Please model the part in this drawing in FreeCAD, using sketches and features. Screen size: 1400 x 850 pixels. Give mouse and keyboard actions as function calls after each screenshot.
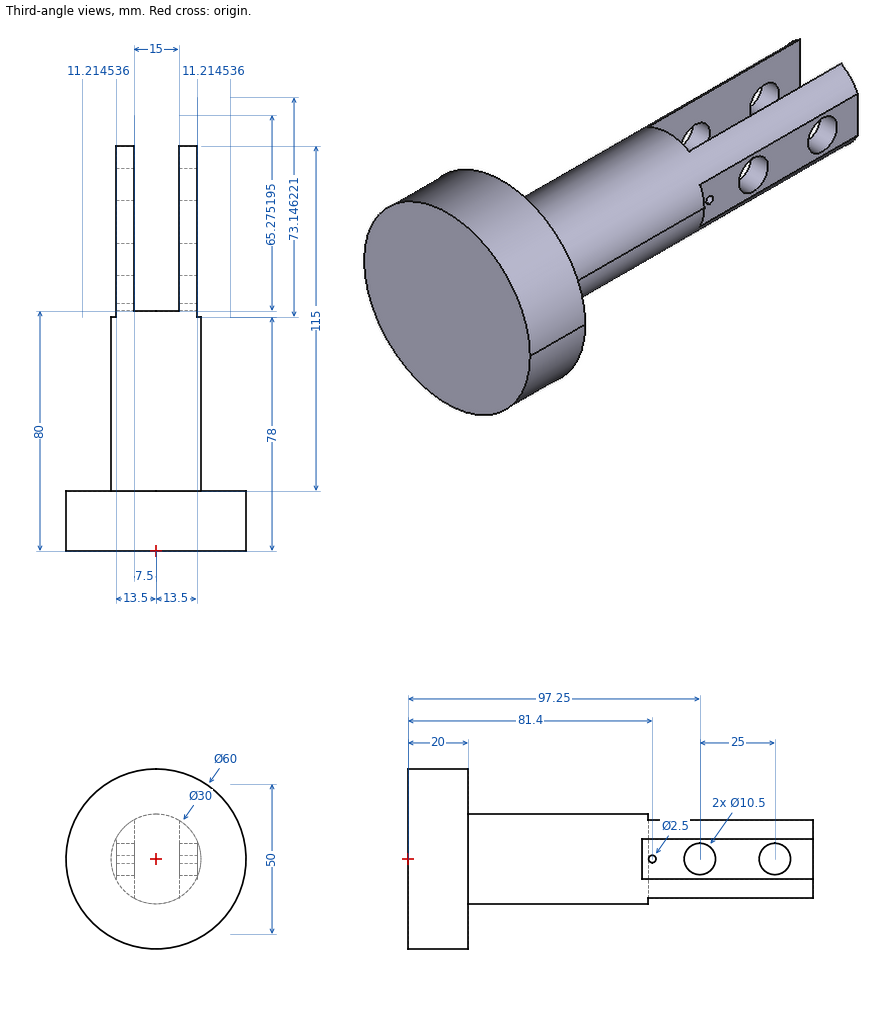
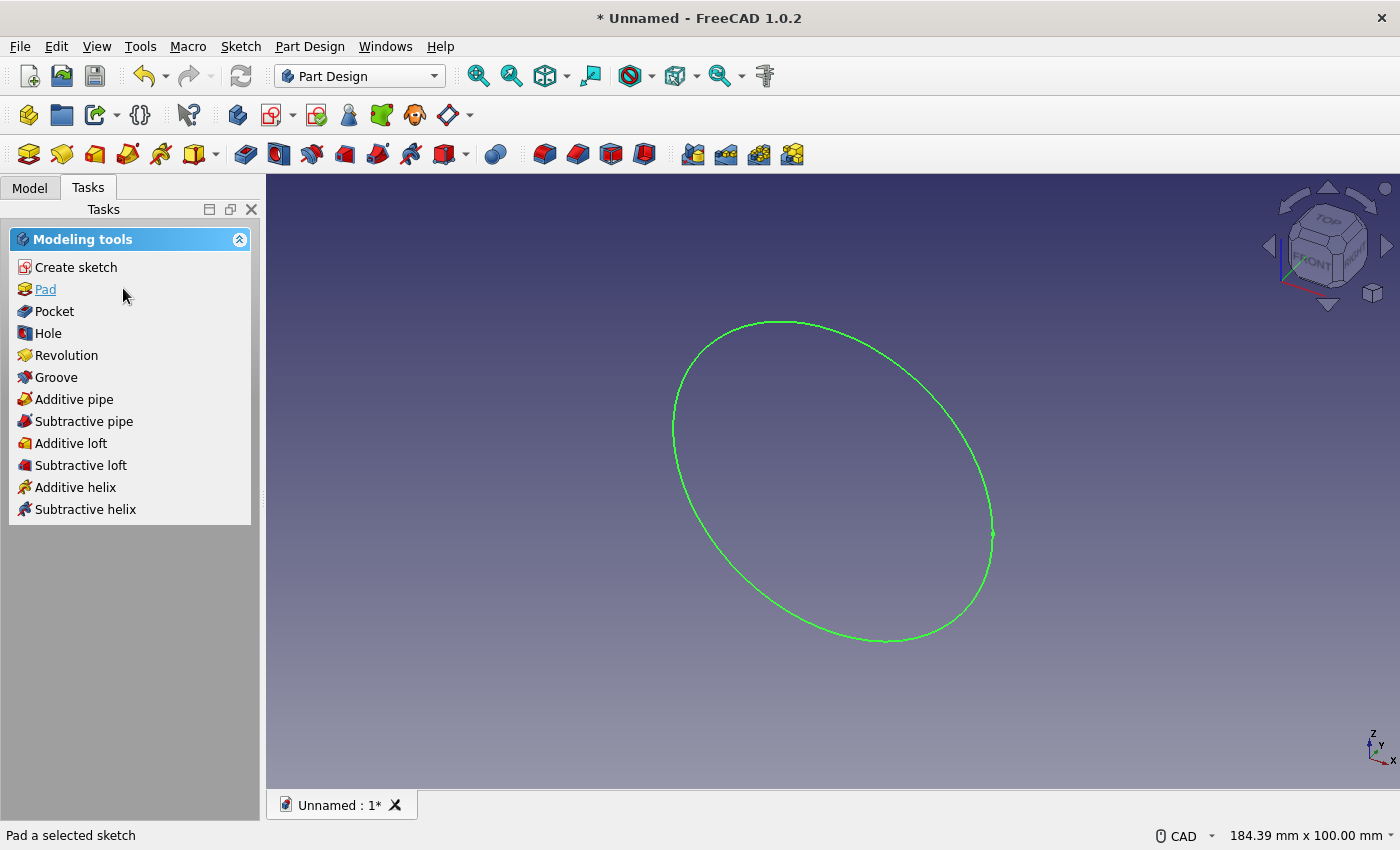
click(29, 154)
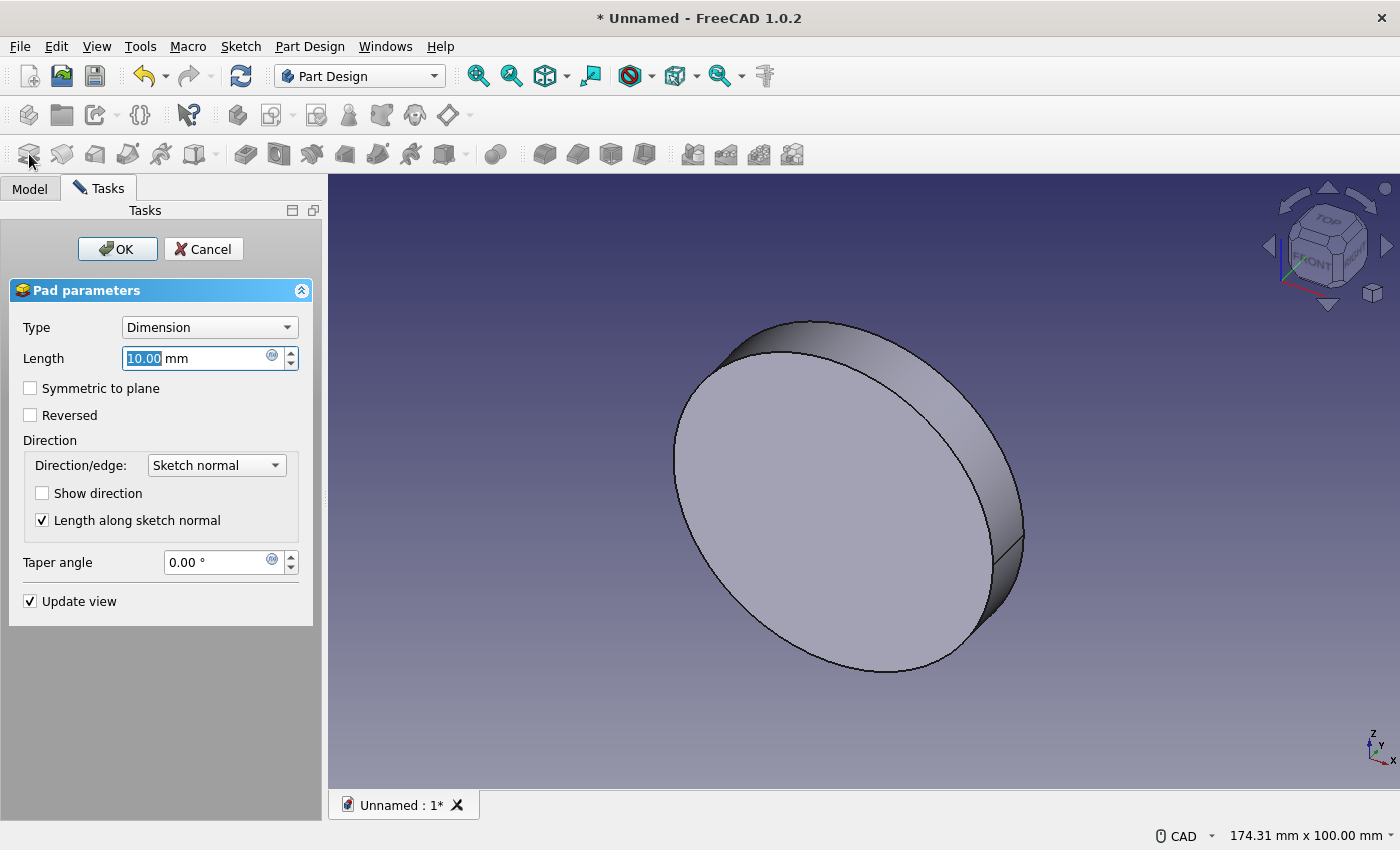
text(20)
key(Tab)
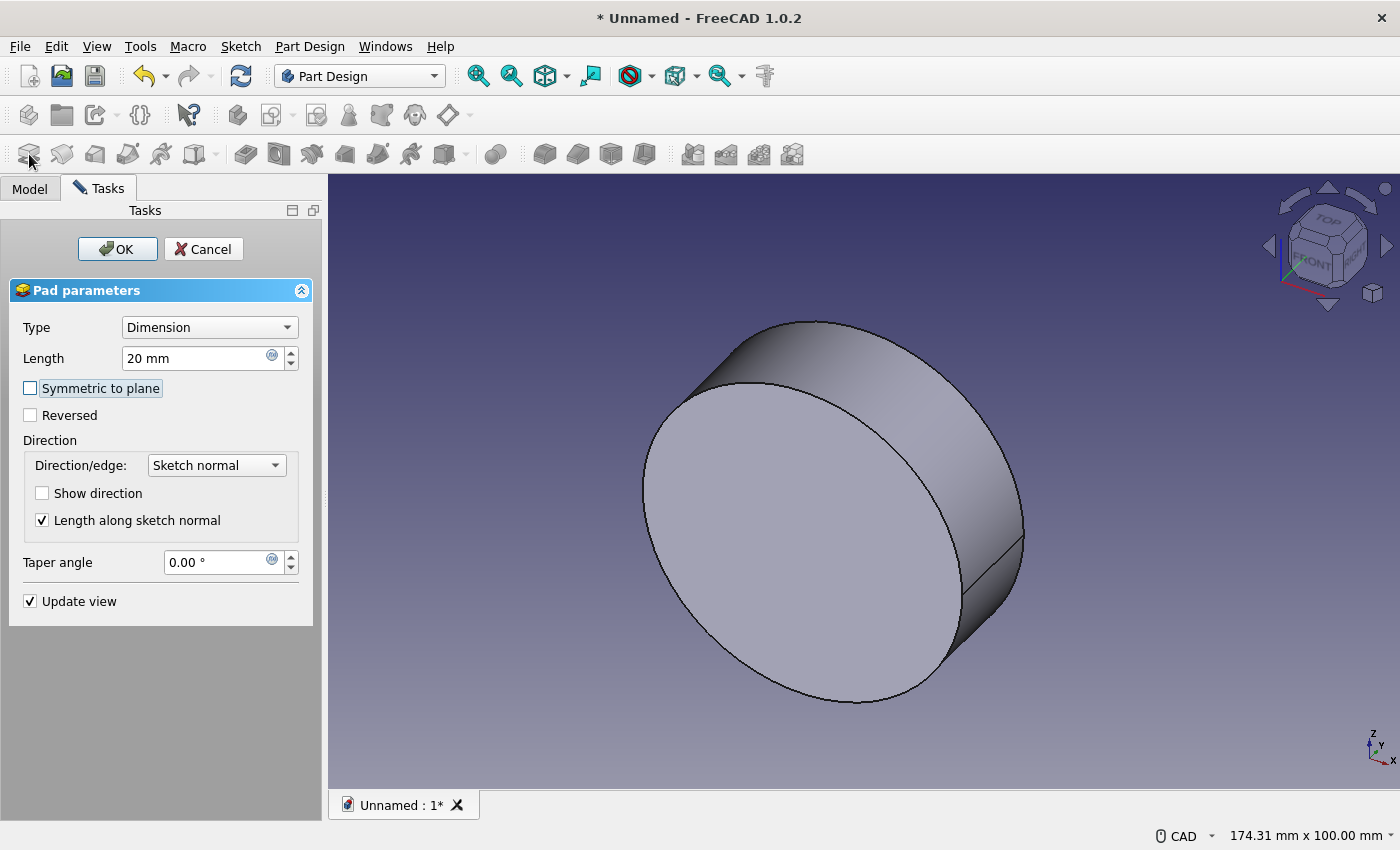
click(31, 415)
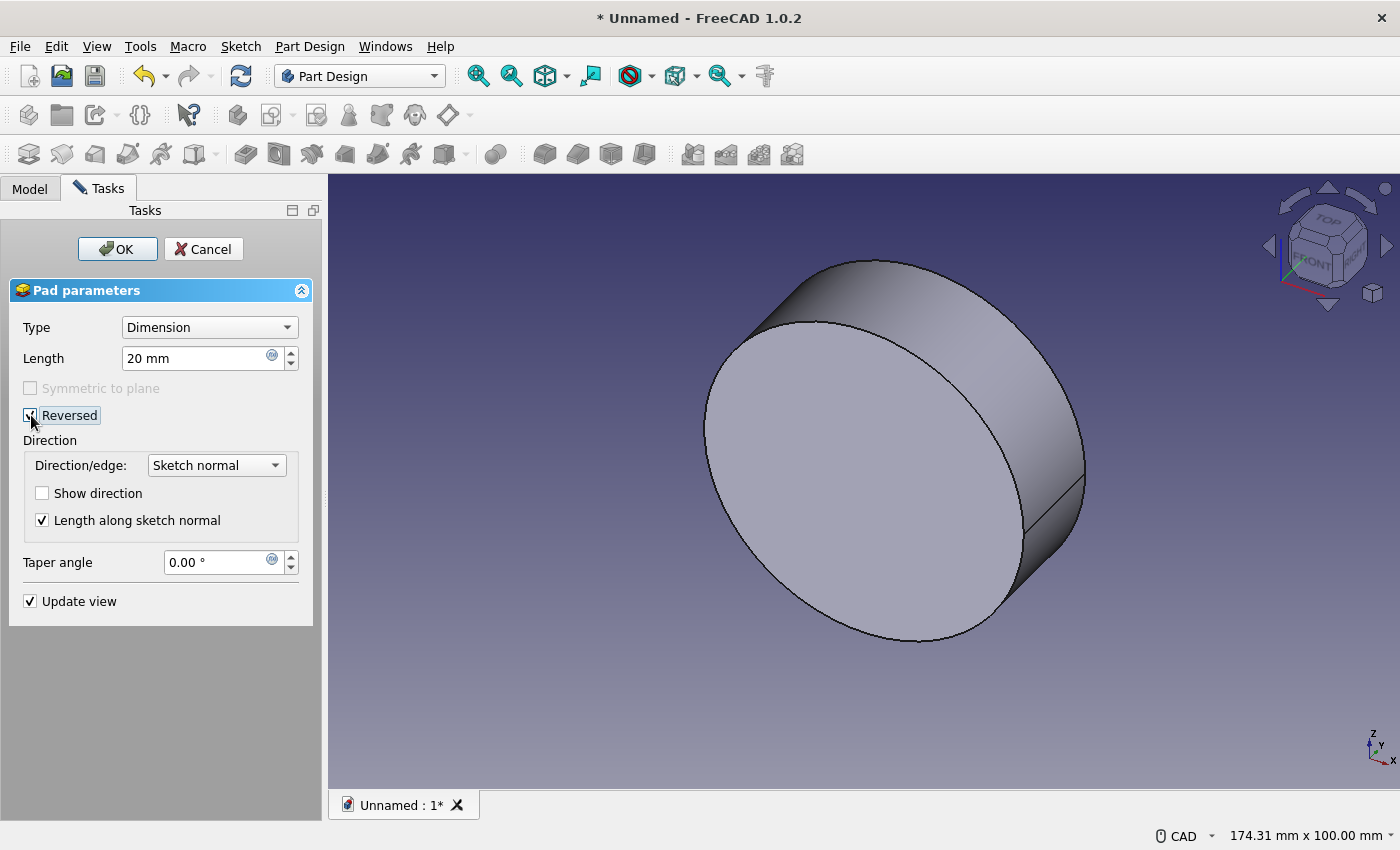
click(118, 249)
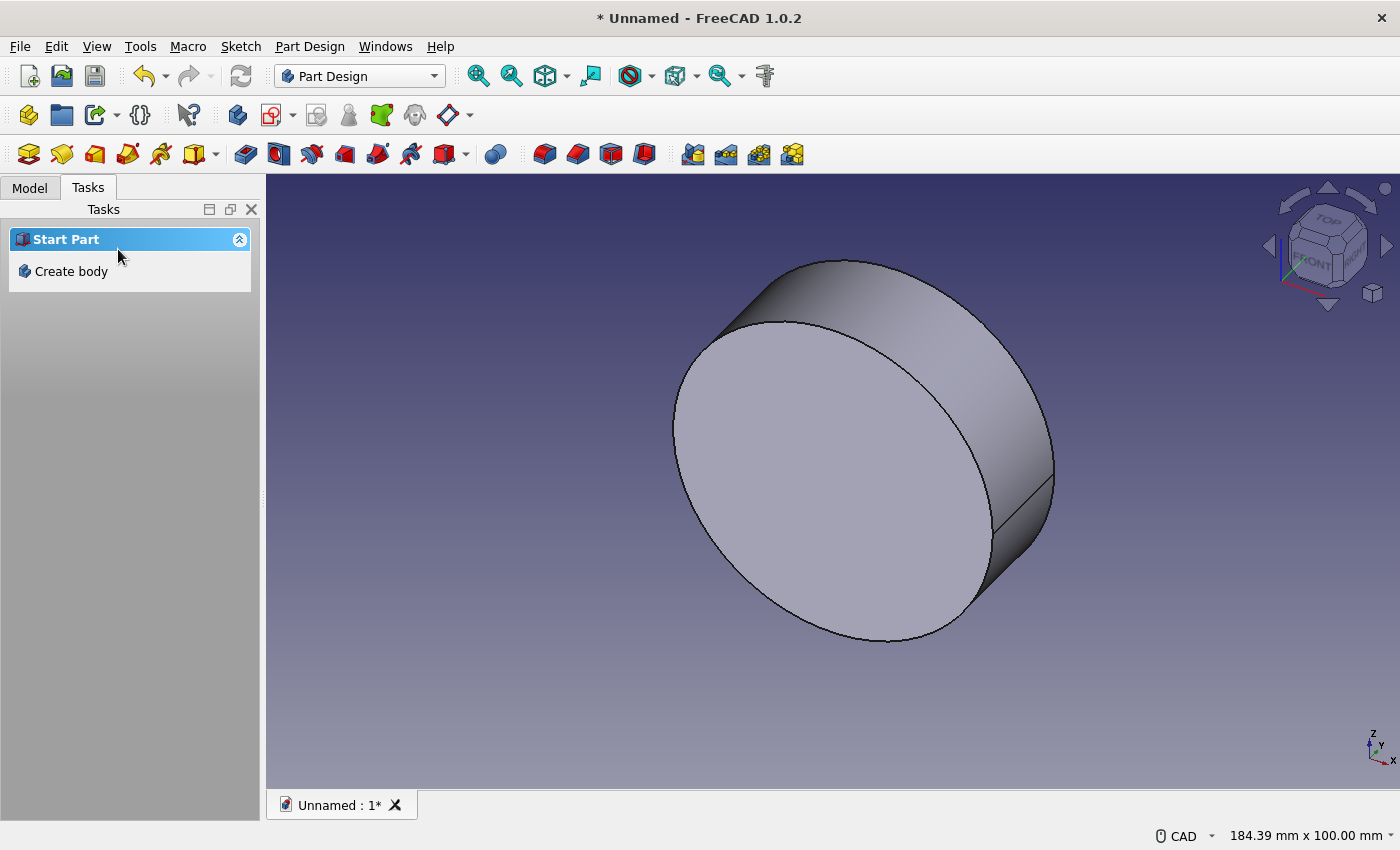
key(4)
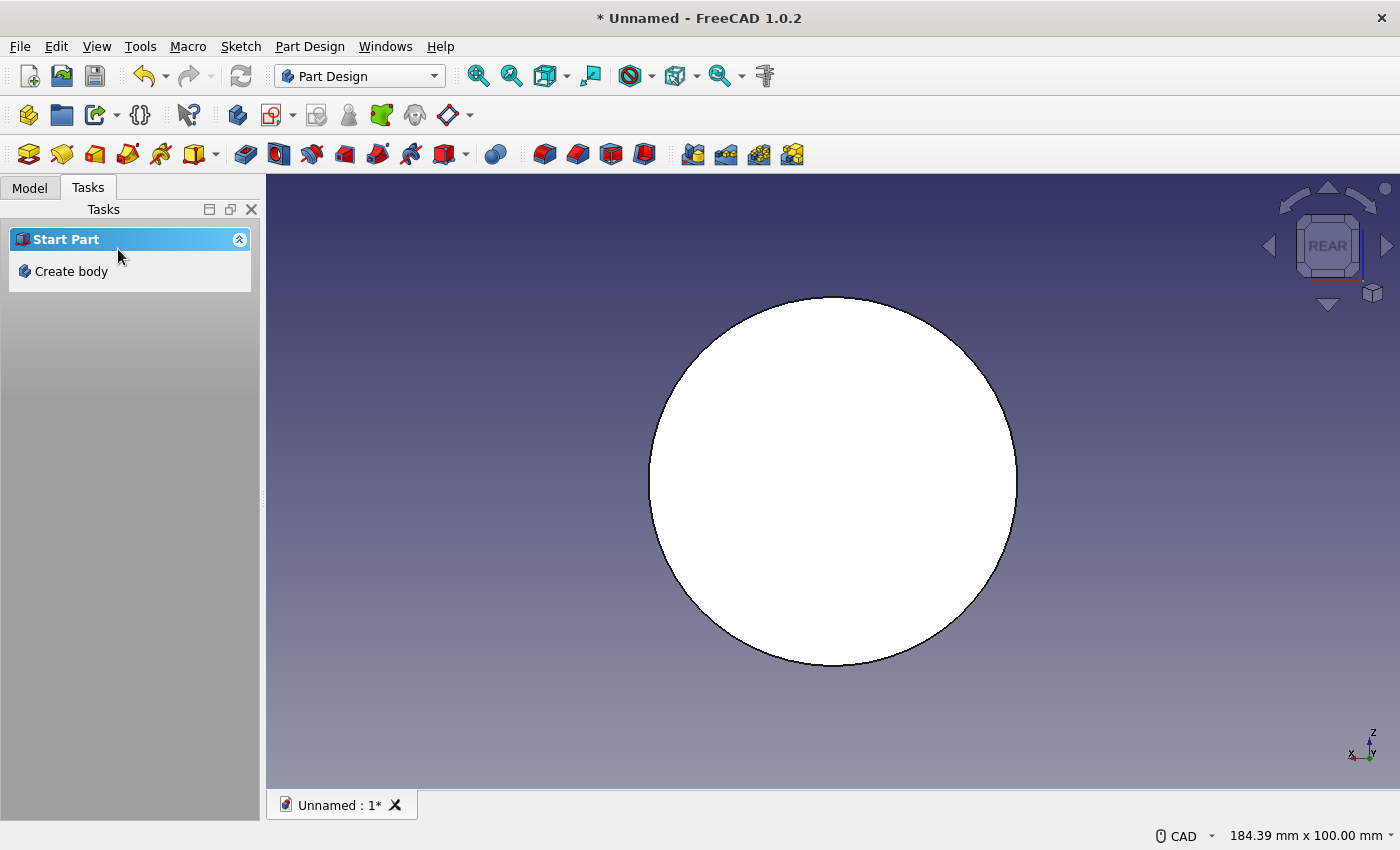
click(833, 480)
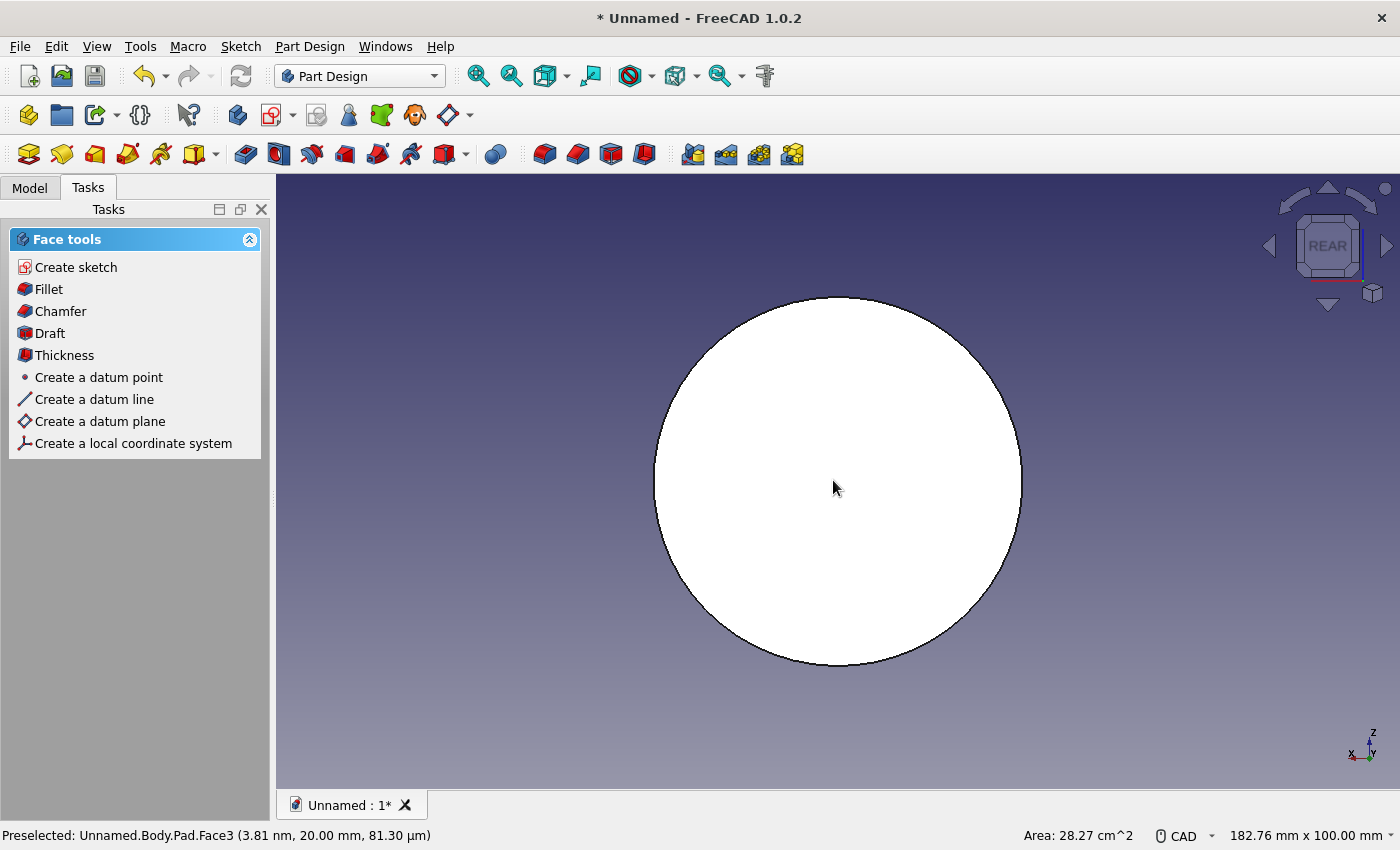
click(270, 116)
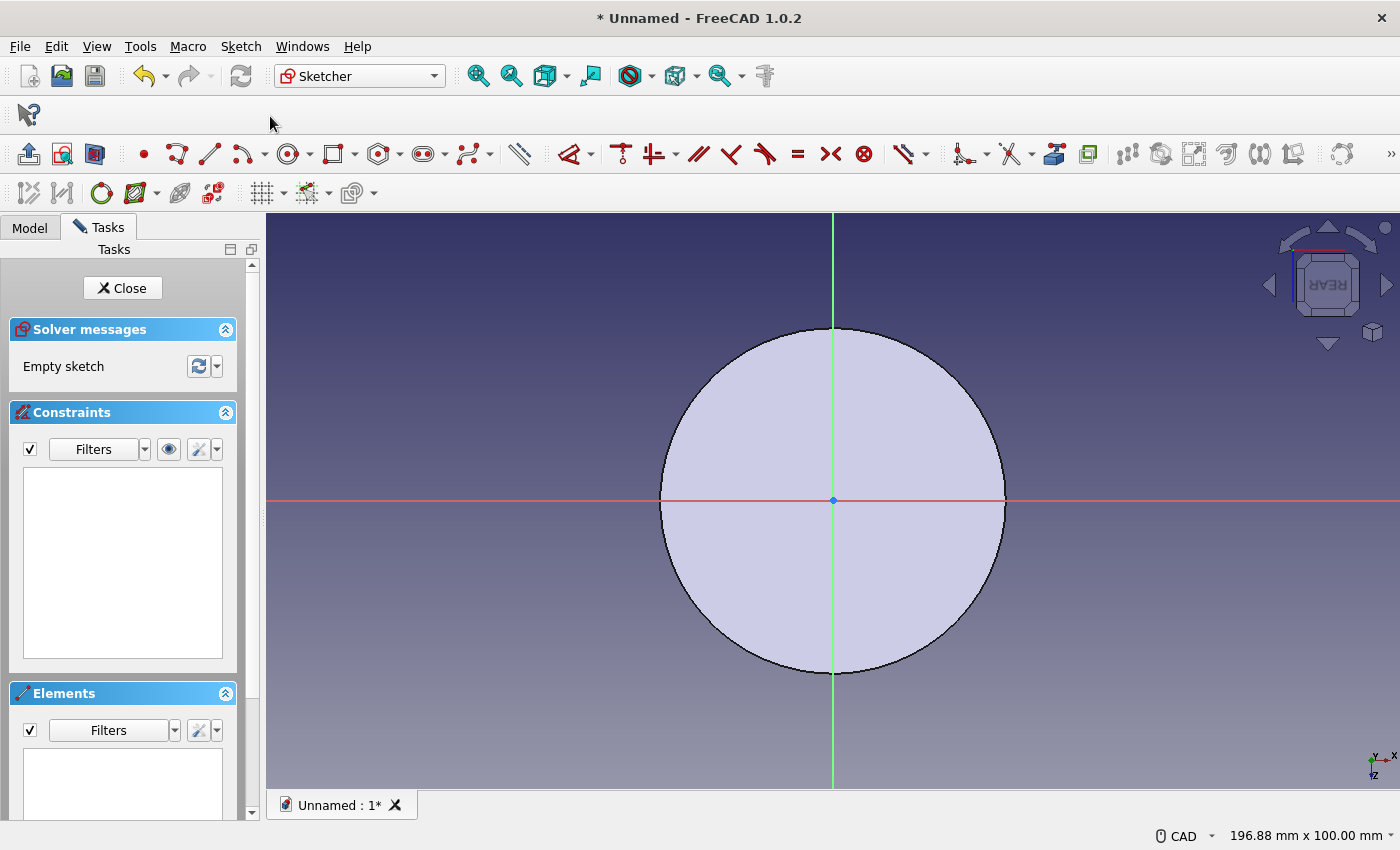
scroll(889, 501, up, 4)